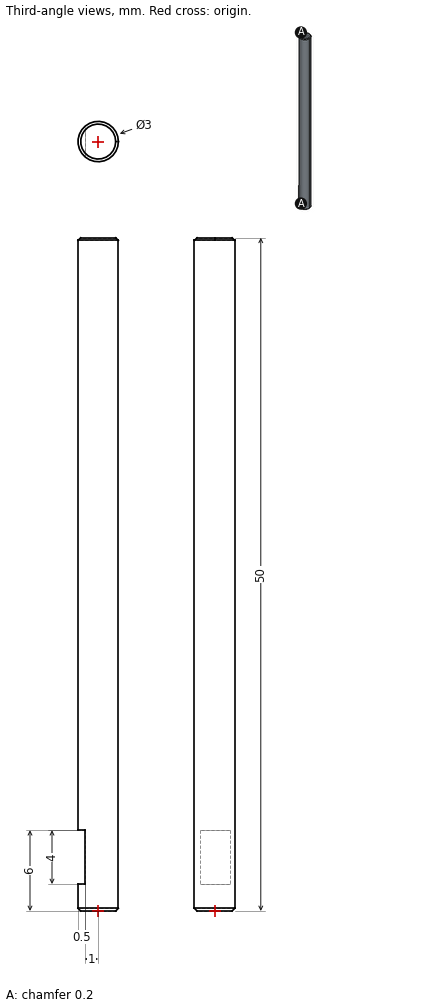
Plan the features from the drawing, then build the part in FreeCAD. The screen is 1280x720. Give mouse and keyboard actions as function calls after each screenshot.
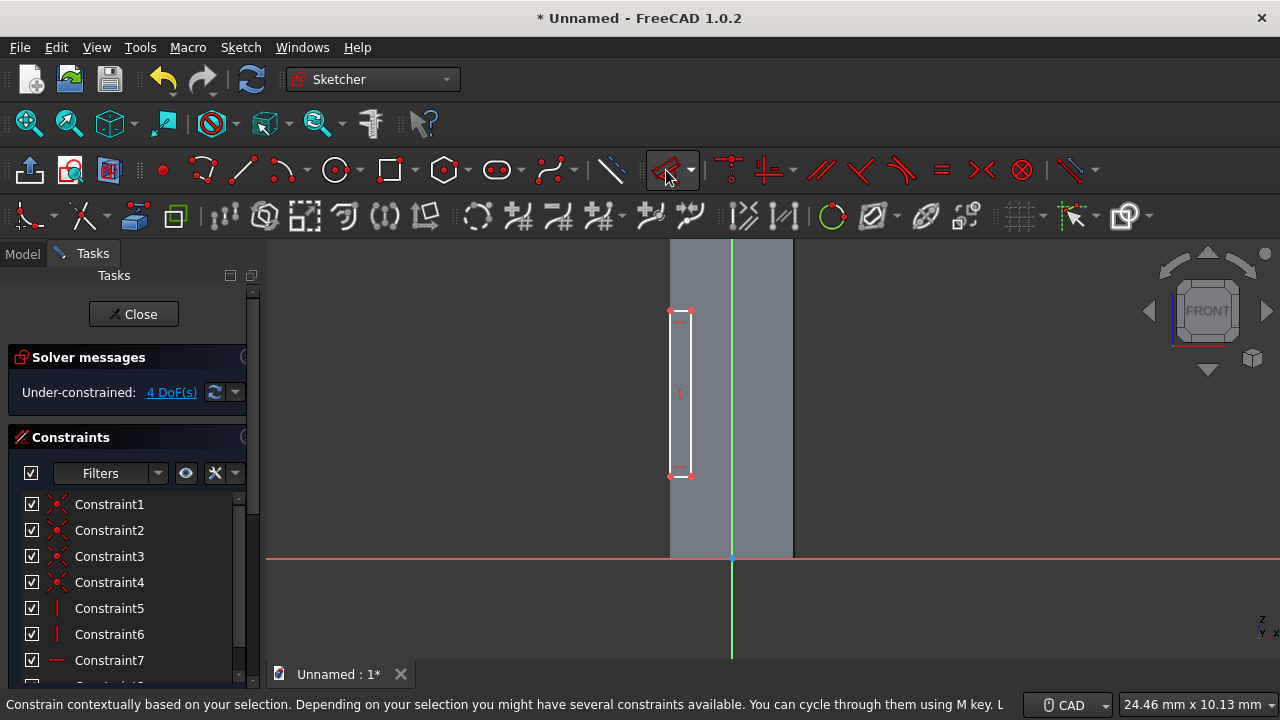
click(670, 361)
click(636, 394)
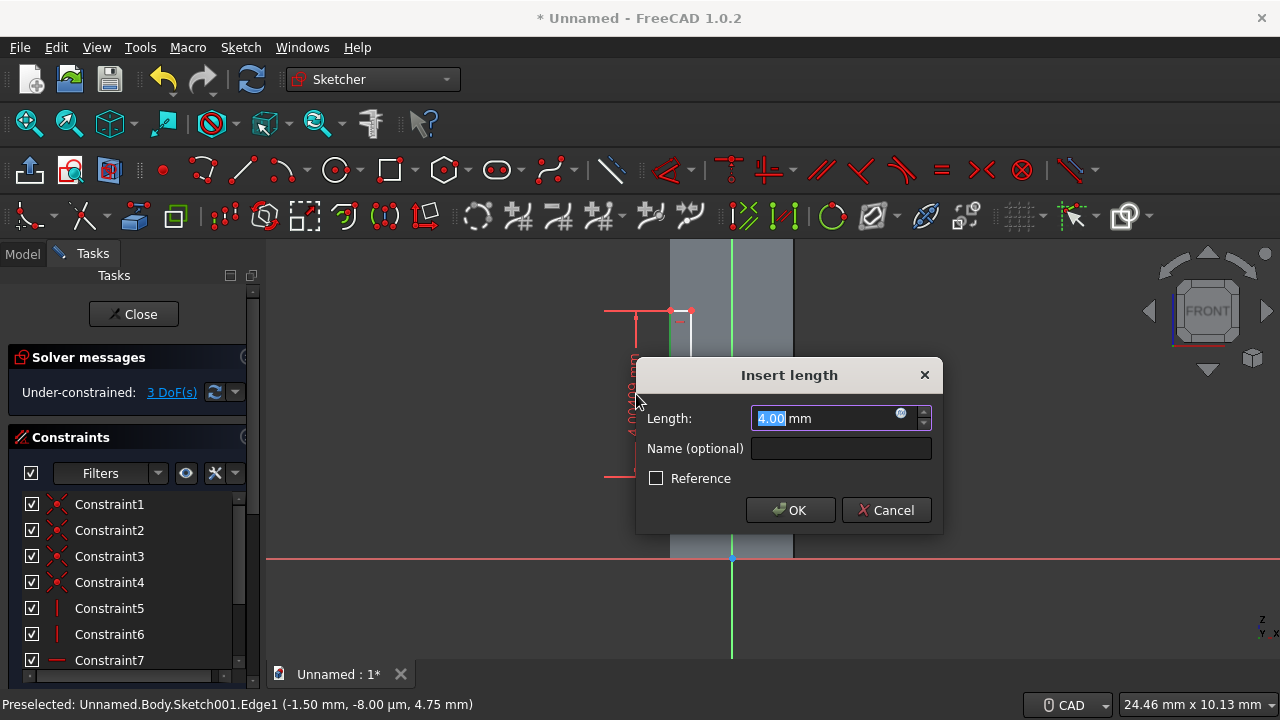
text(4)
key(Return)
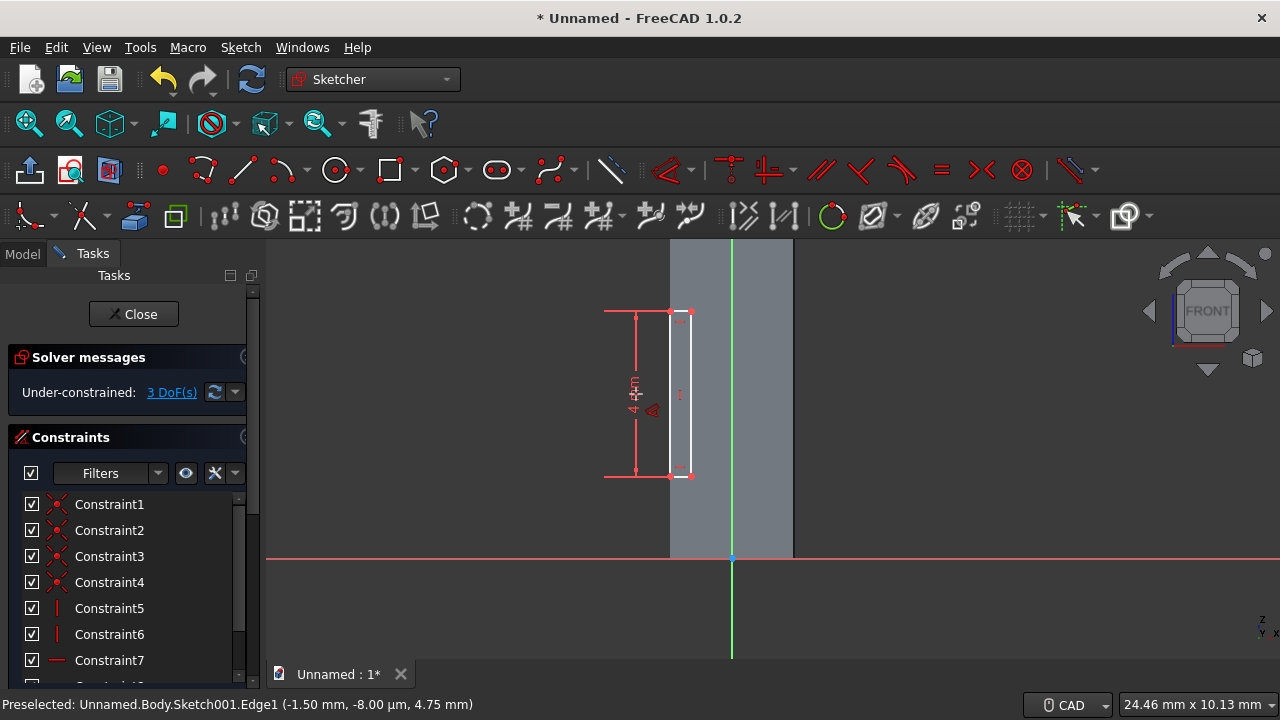
click(670, 311)
click(766, 435)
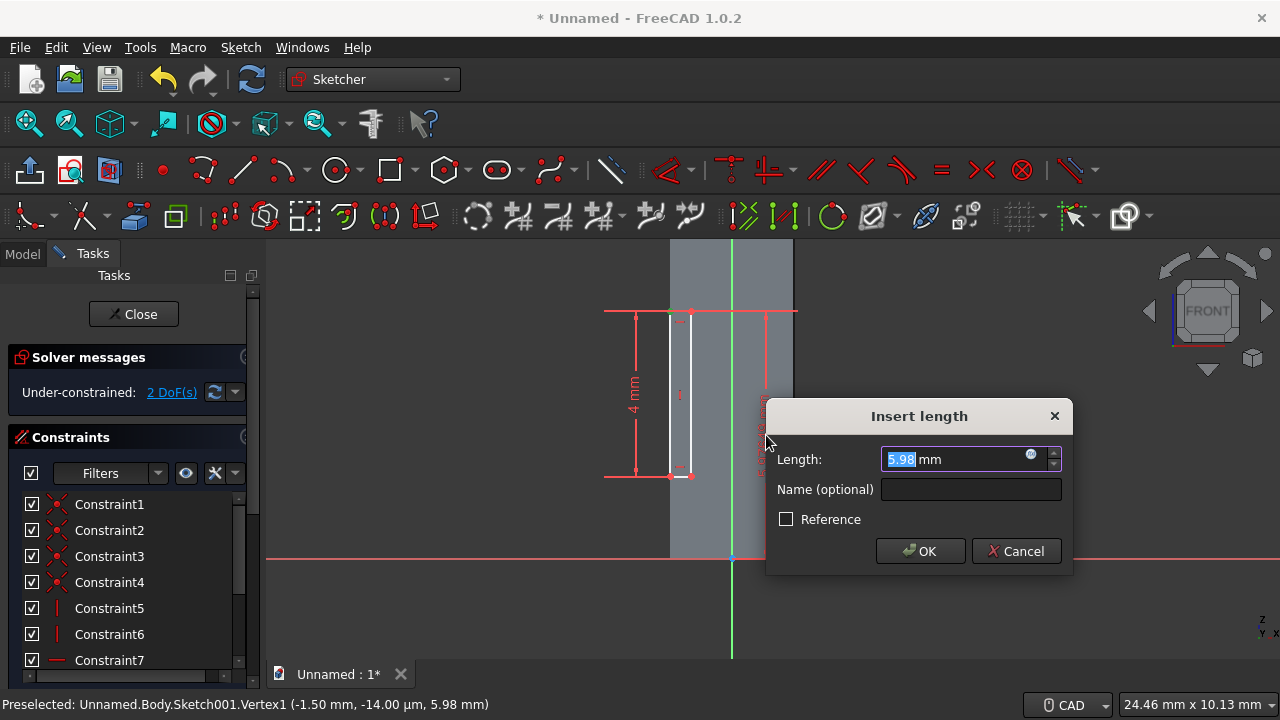
text(6)
key(Return)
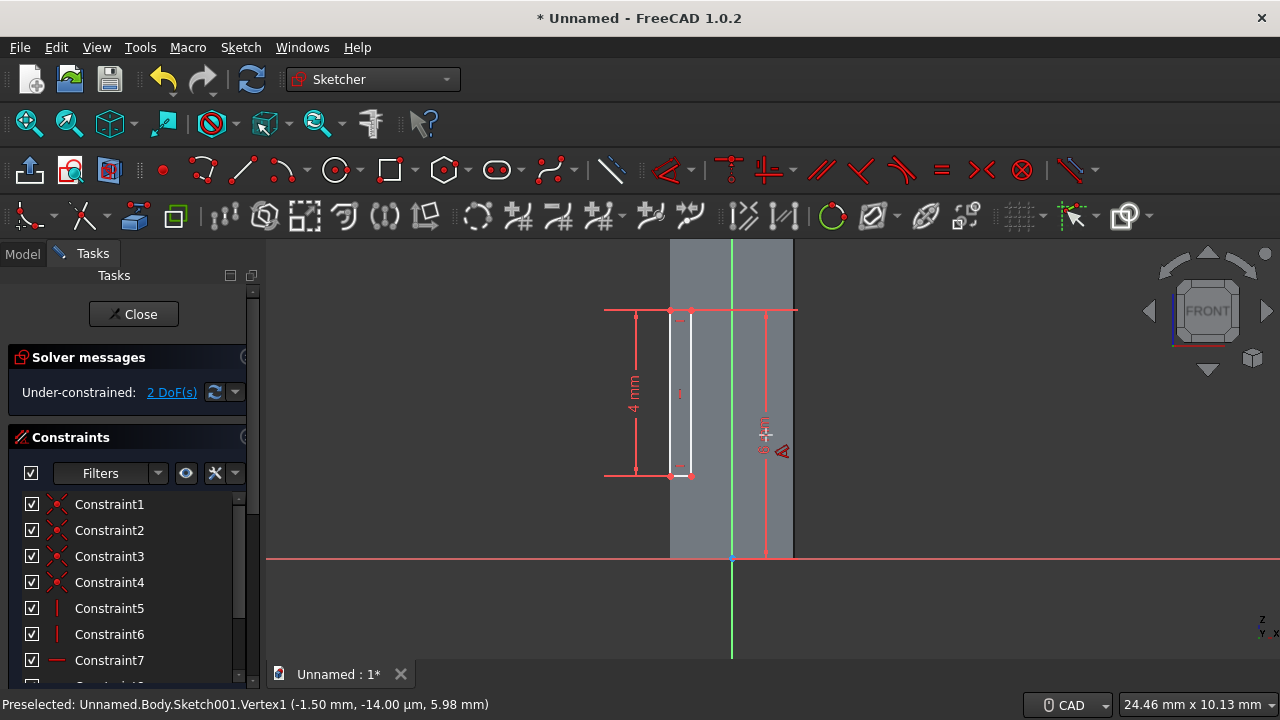
click(691, 476)
click(712, 593)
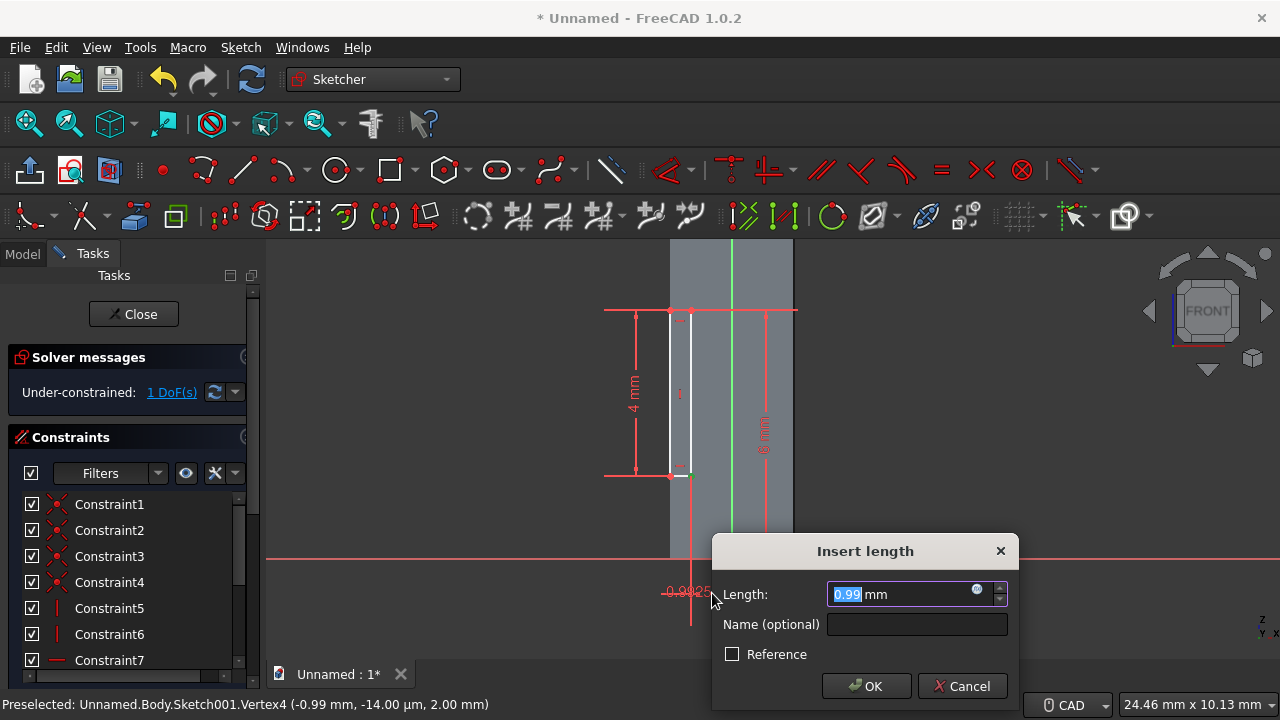
text(1)
key(Return)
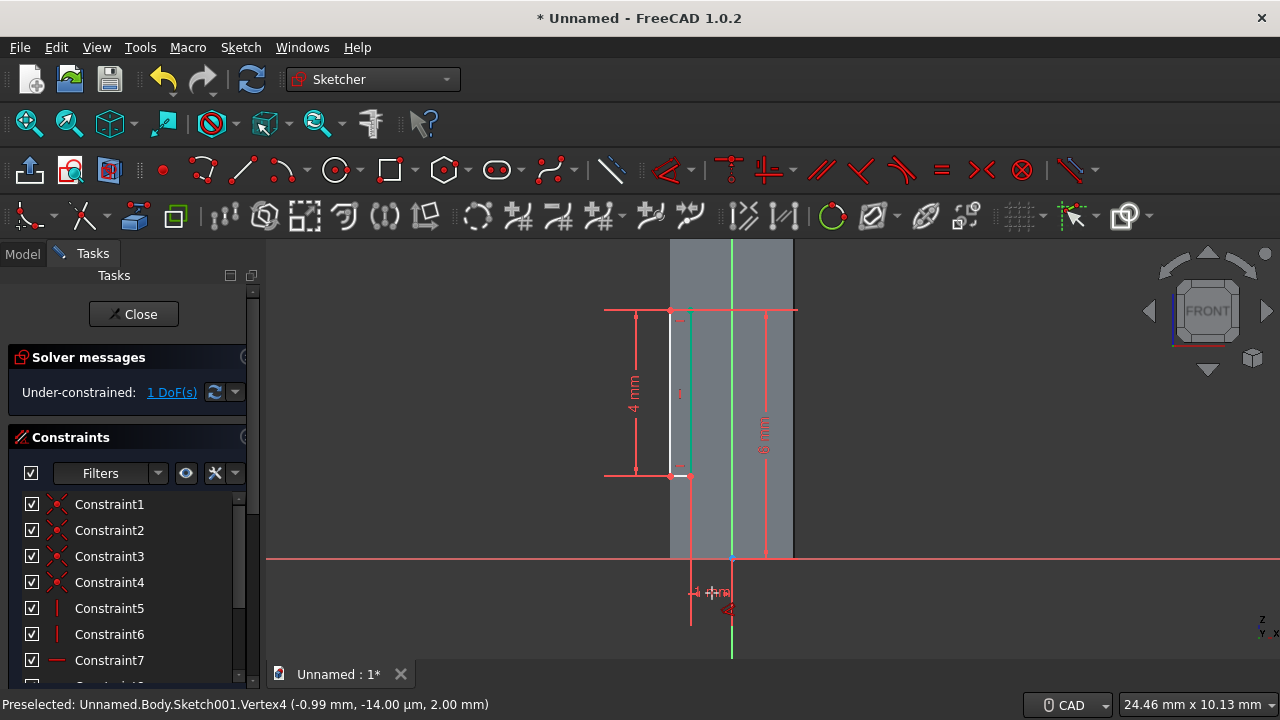
scroll(680, 476, up, 4)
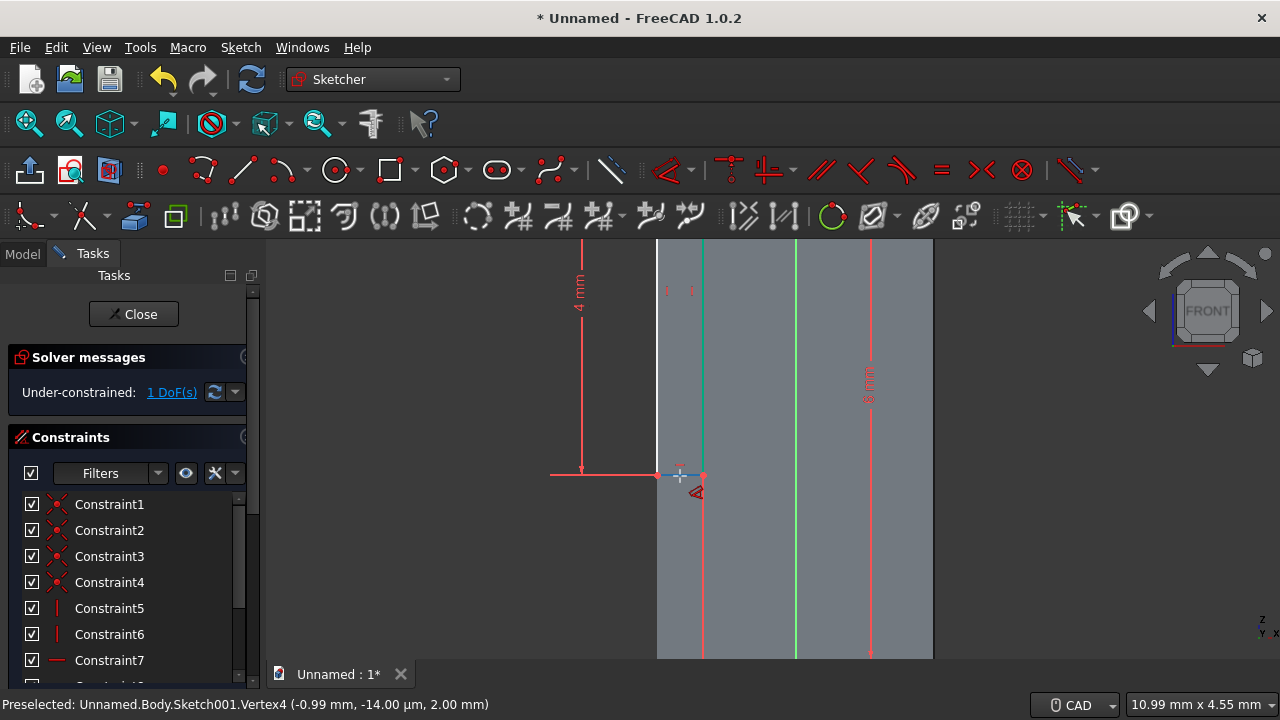
click(680, 475)
click(680, 509)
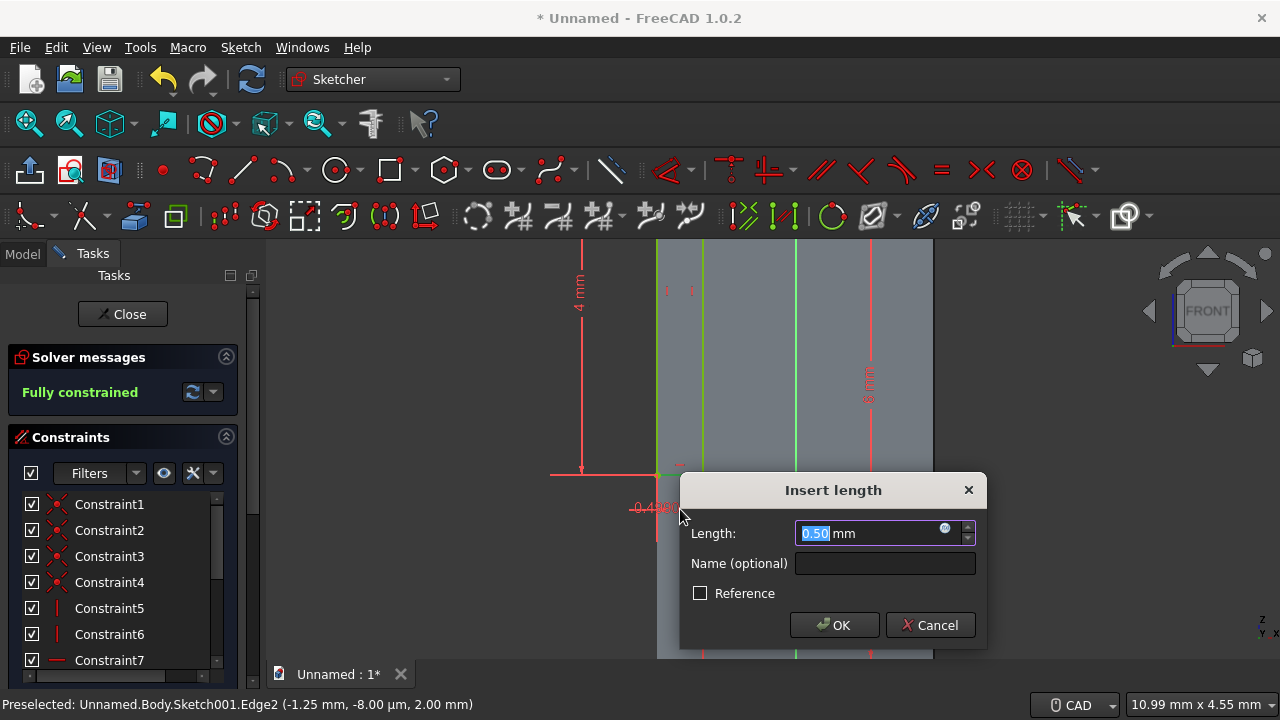
text(0.5)
key(Return)
key(Escape)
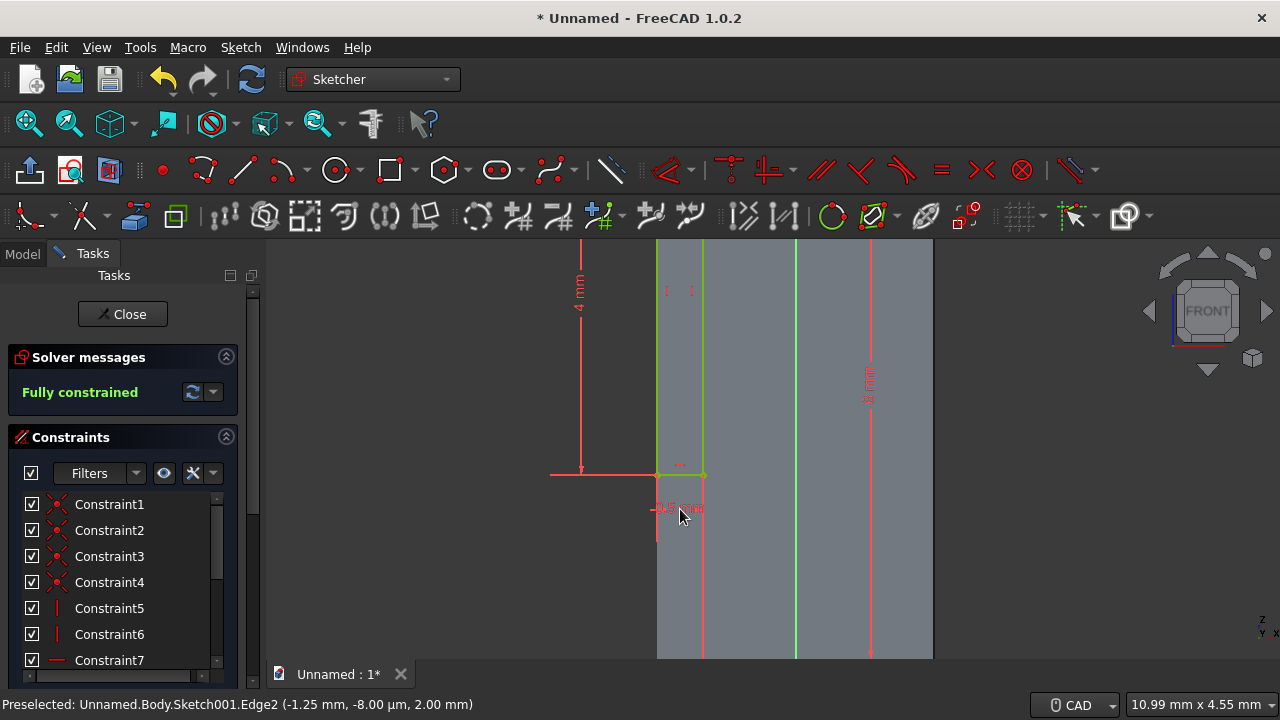
click(123, 314)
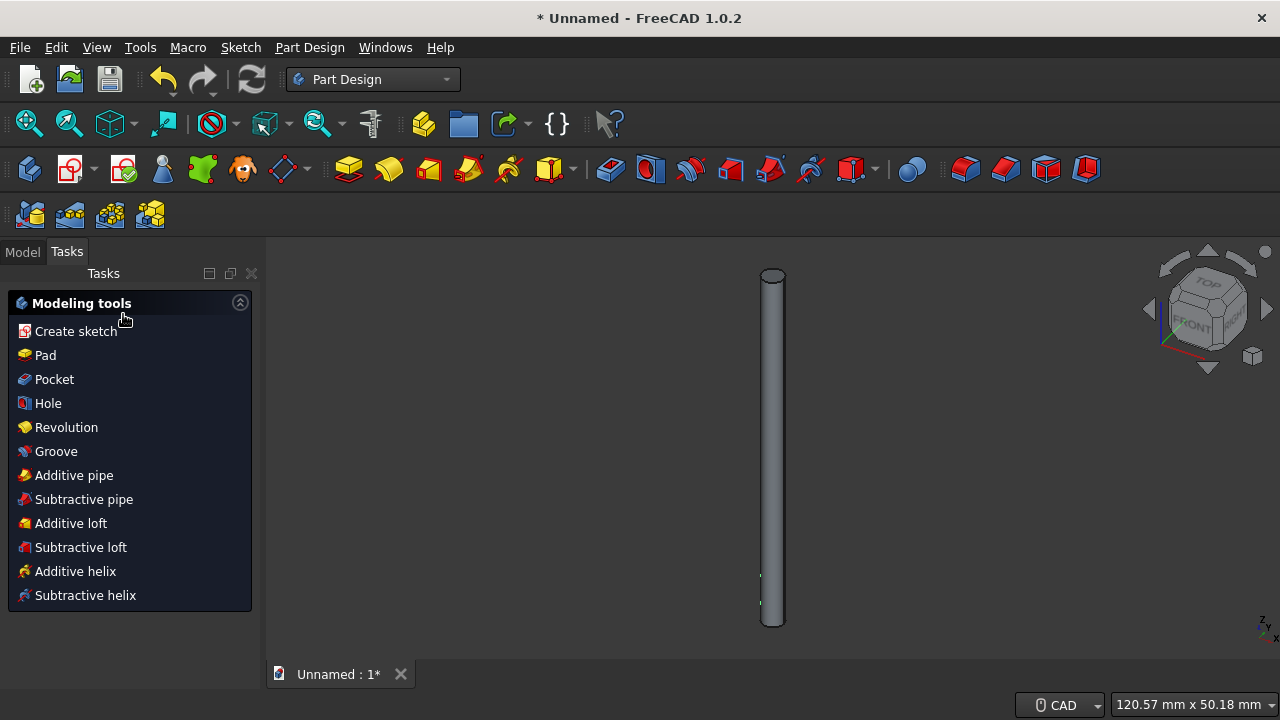
click(612, 170)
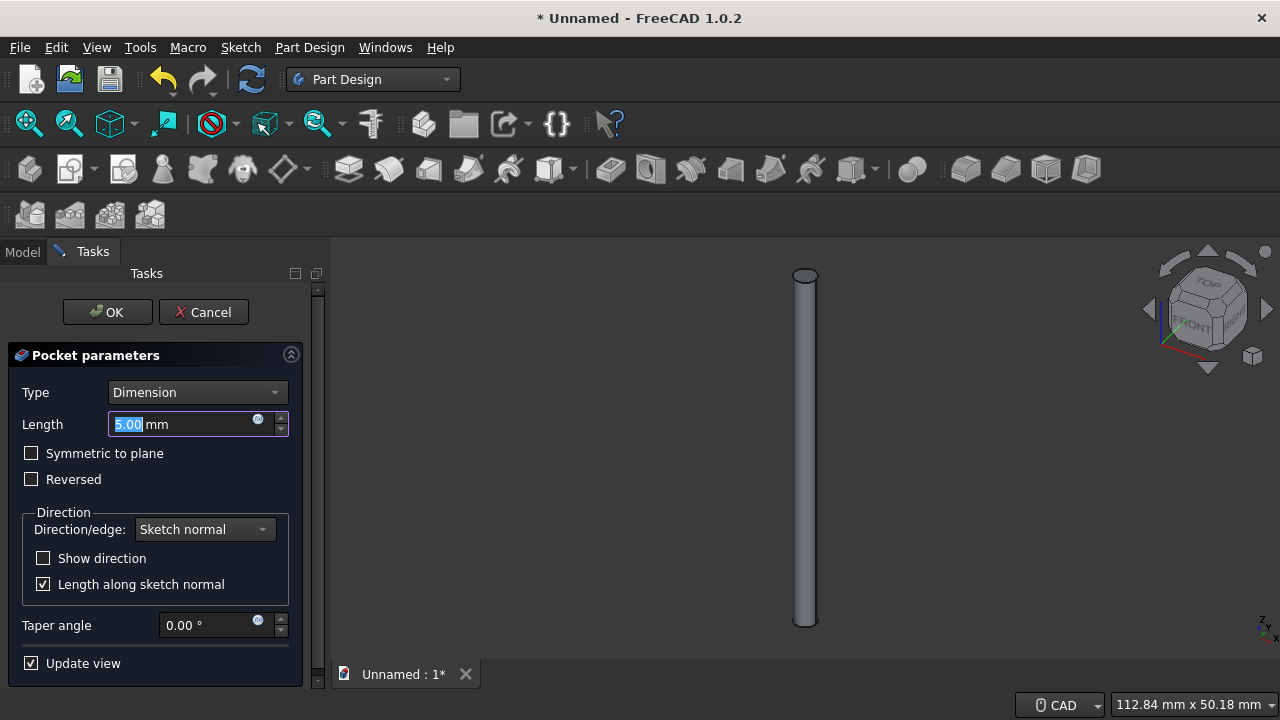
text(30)
key(Tab)